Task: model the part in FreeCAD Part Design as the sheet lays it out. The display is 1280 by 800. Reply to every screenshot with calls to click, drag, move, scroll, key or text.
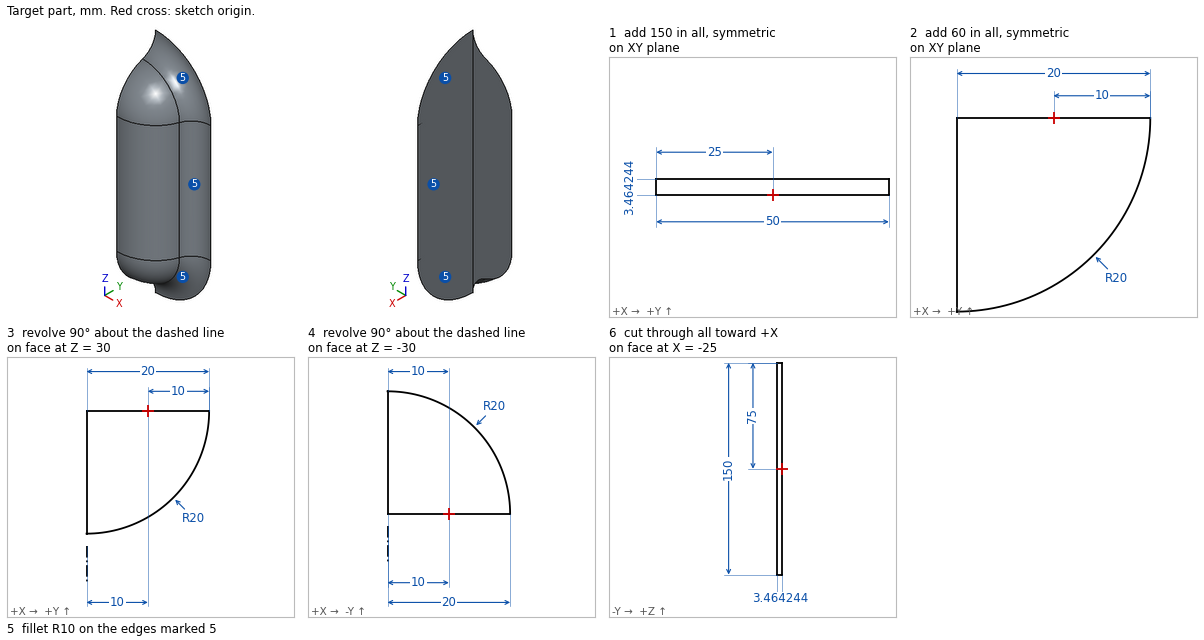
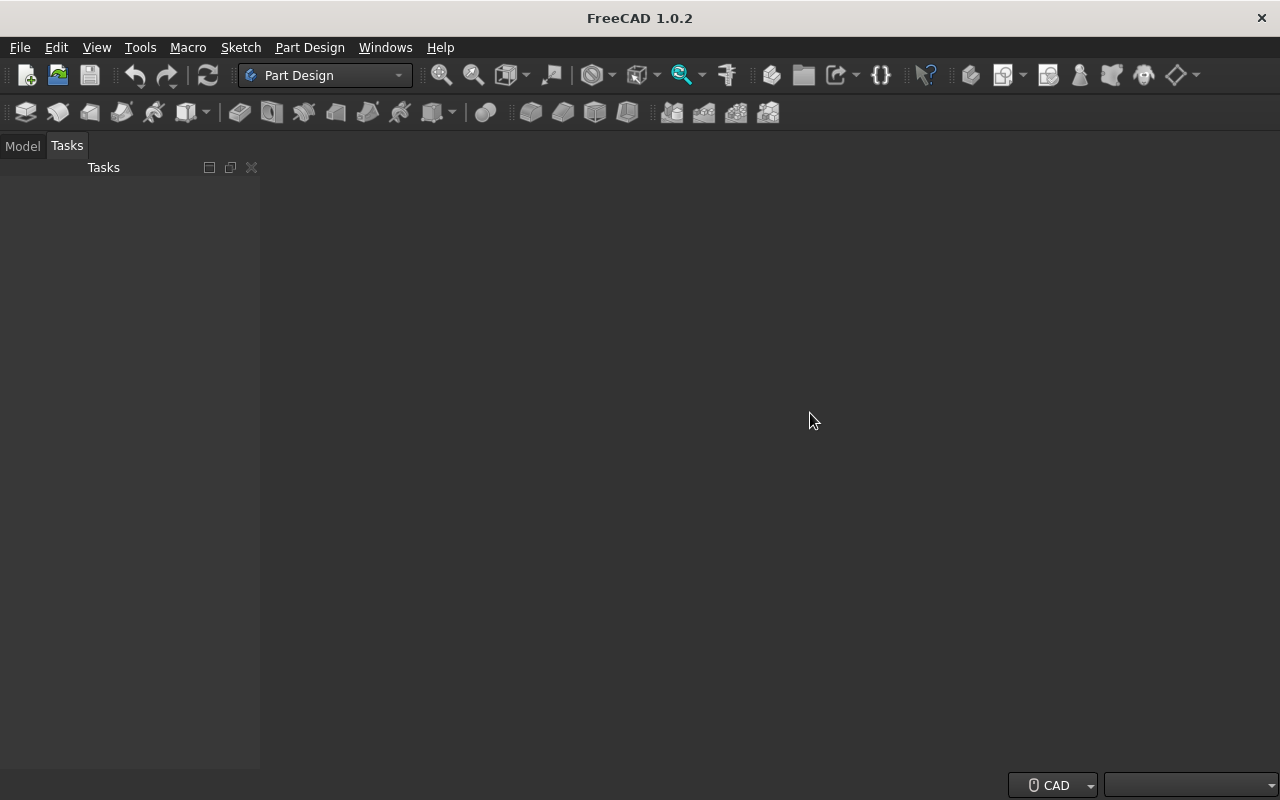
click(26, 76)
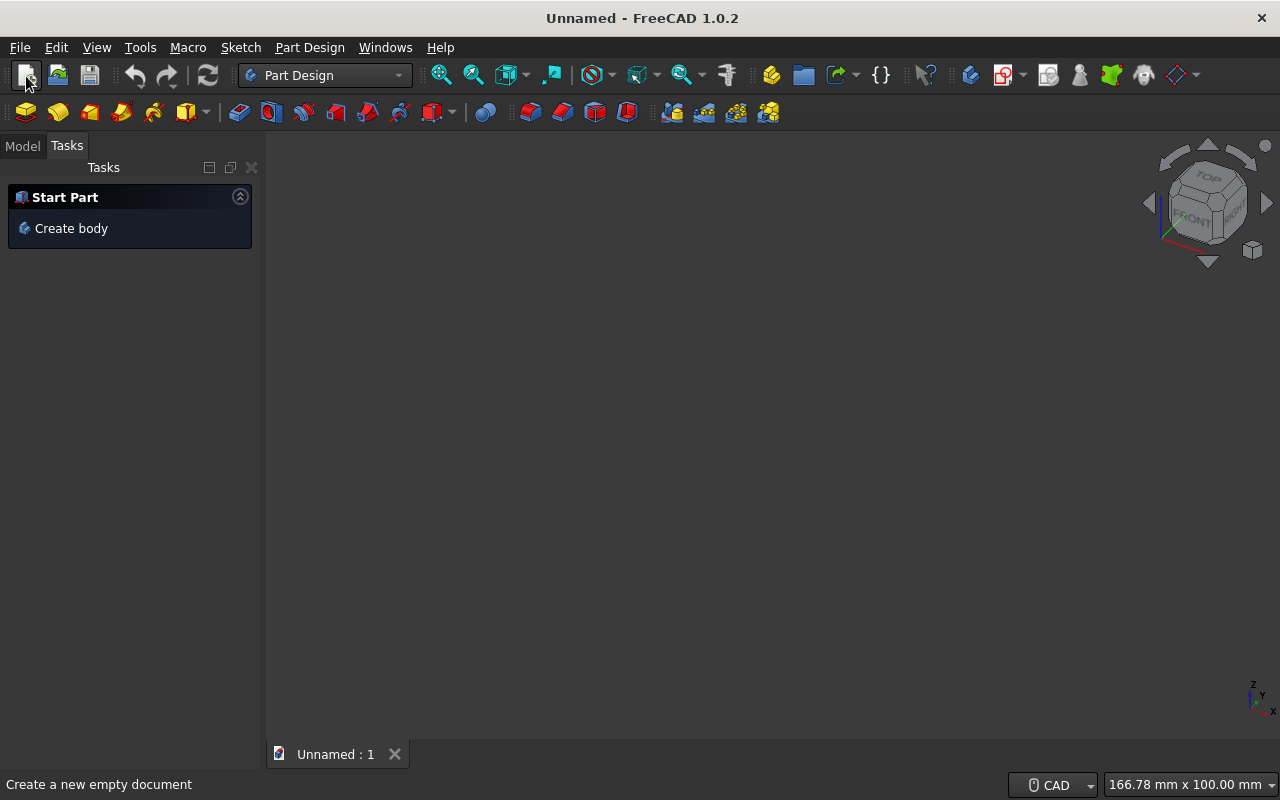
click(1004, 76)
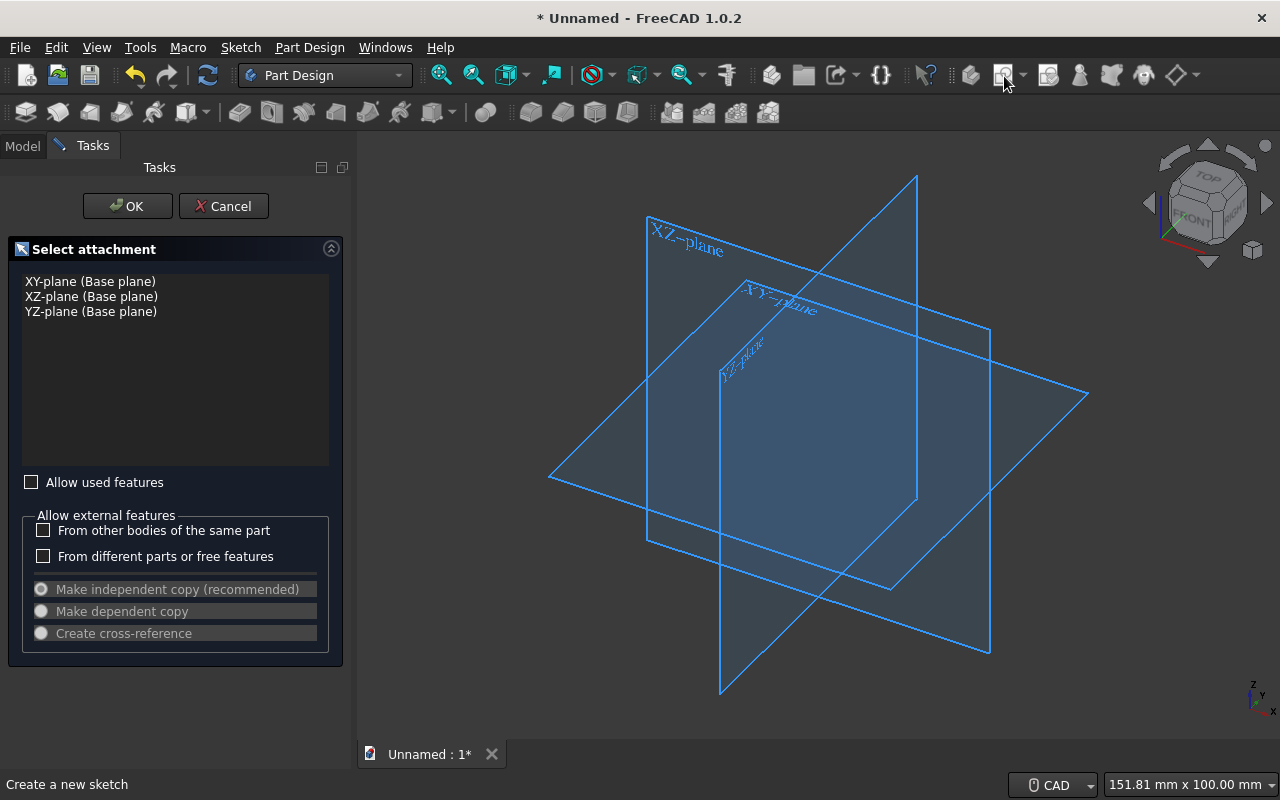
click(82, 282)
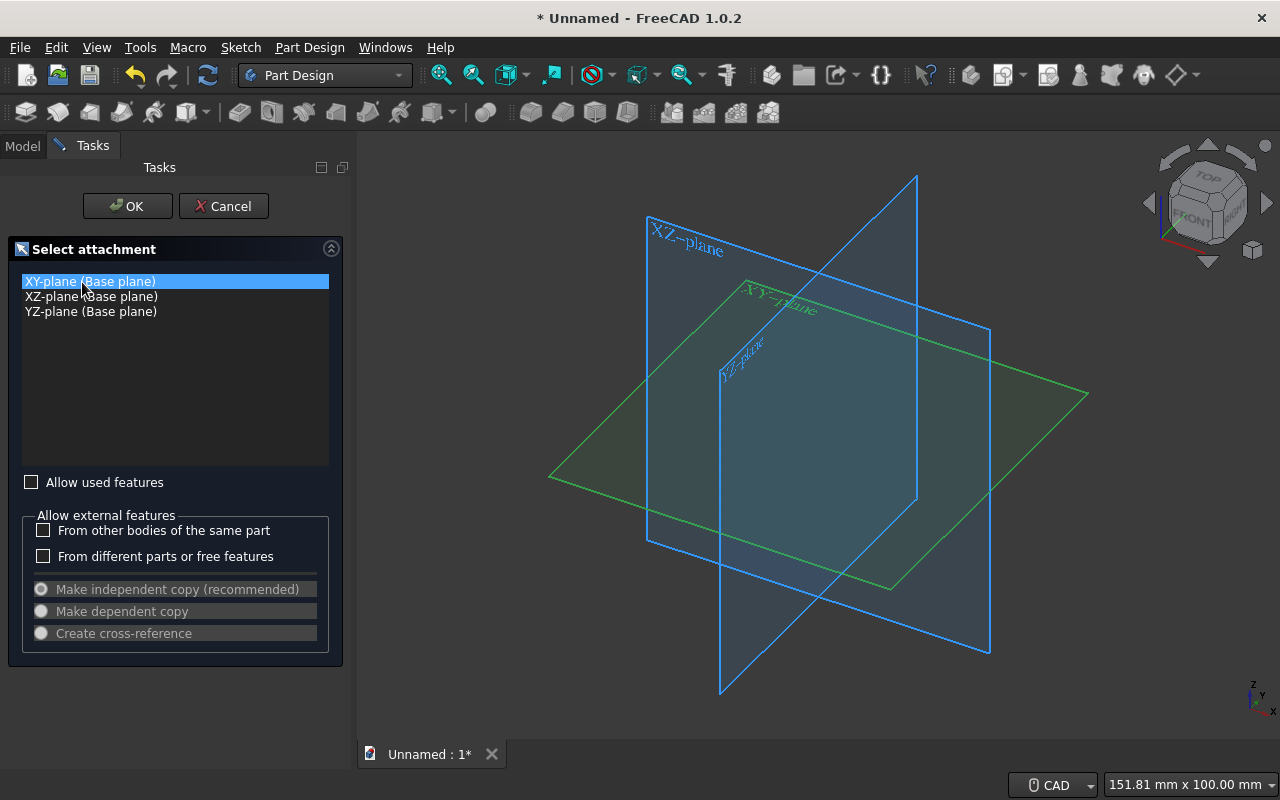
click(128, 206)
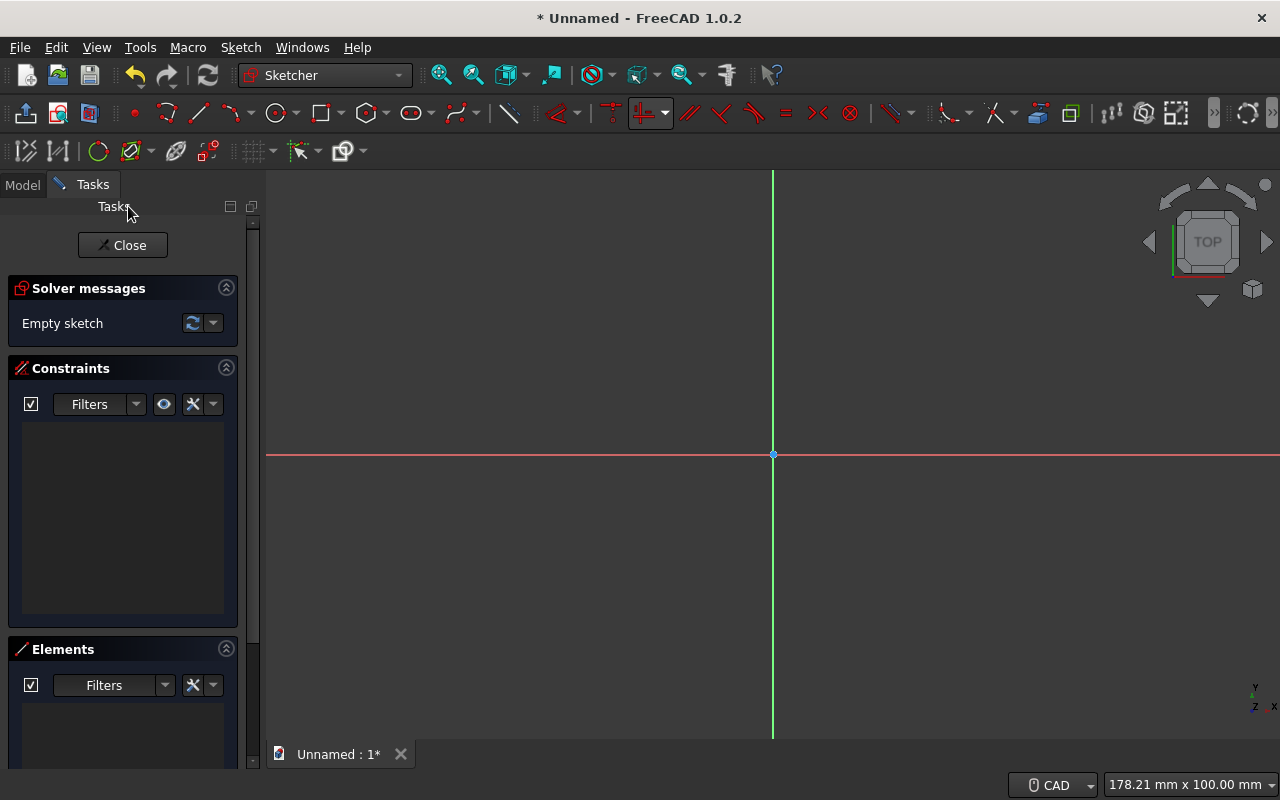
scroll(829, 437, up, 4)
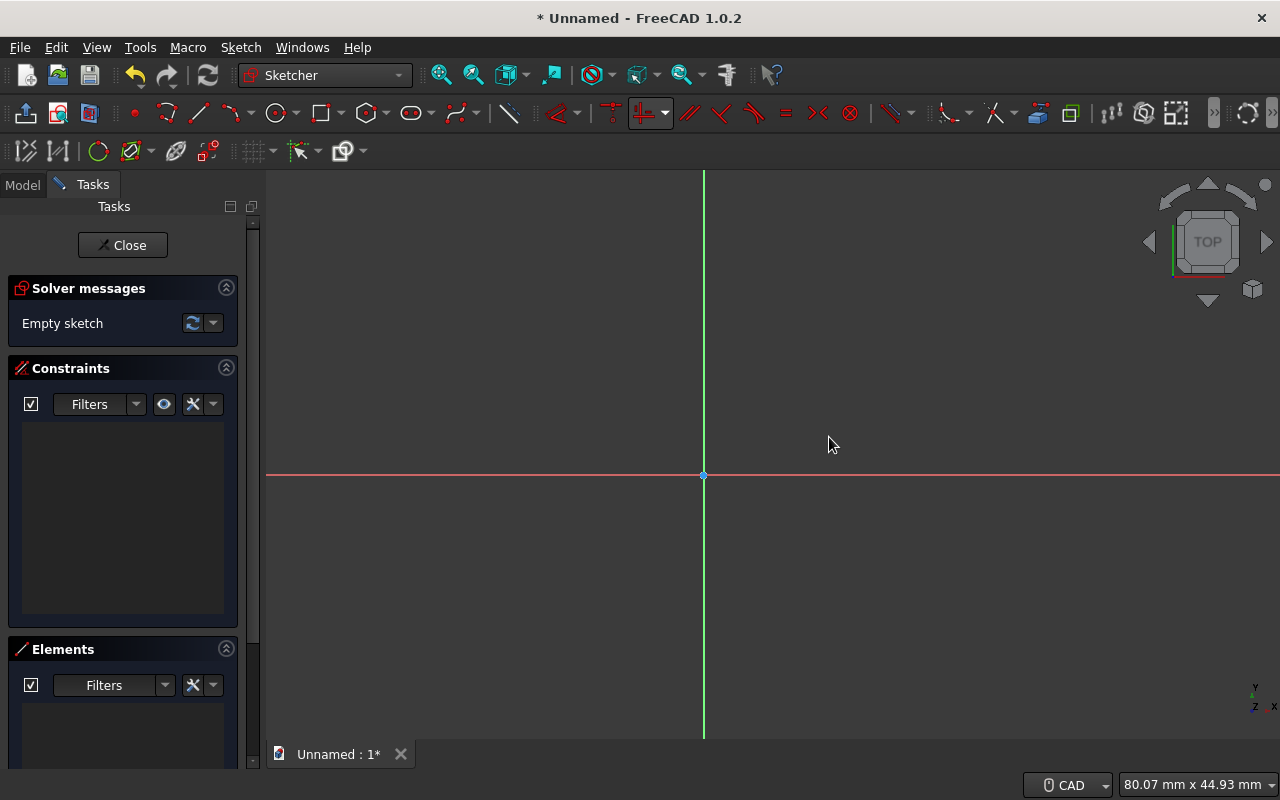
click(322, 114)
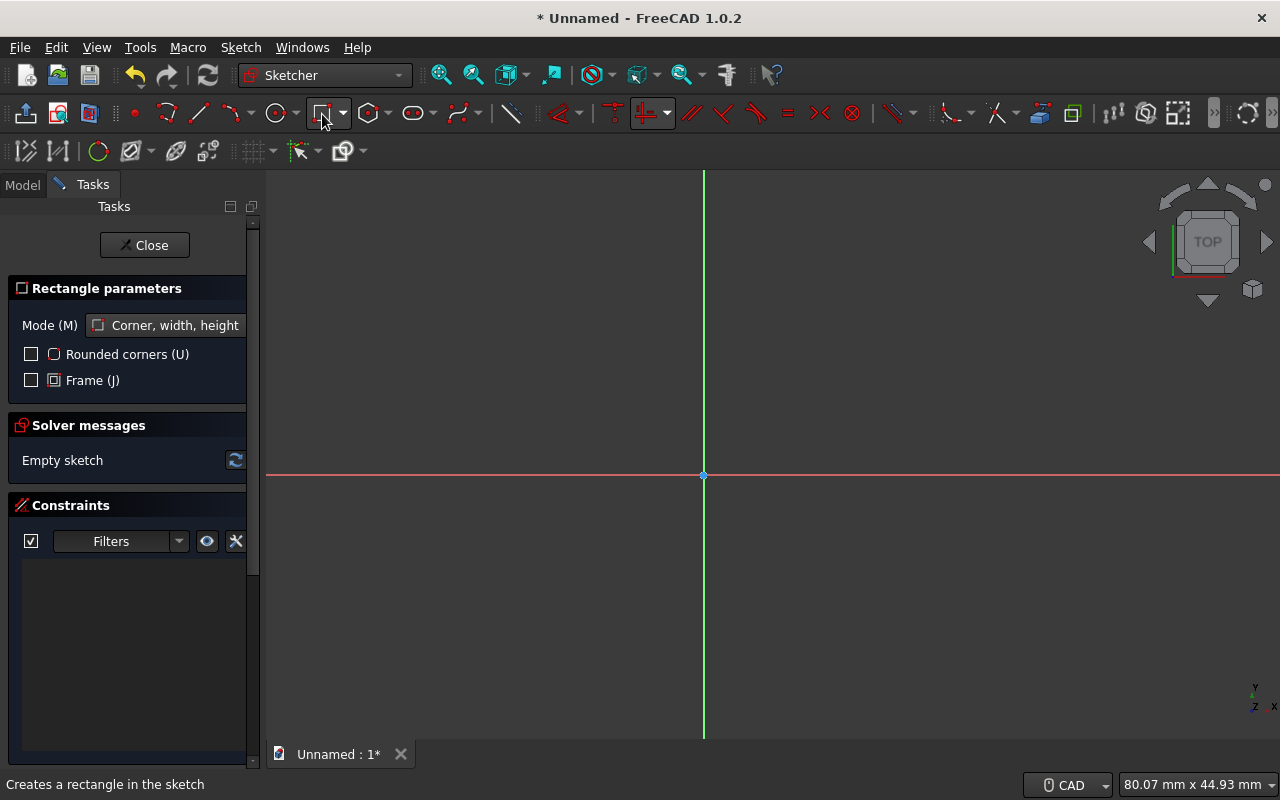
click(387, 432)
click(1020, 475)
key(Escape)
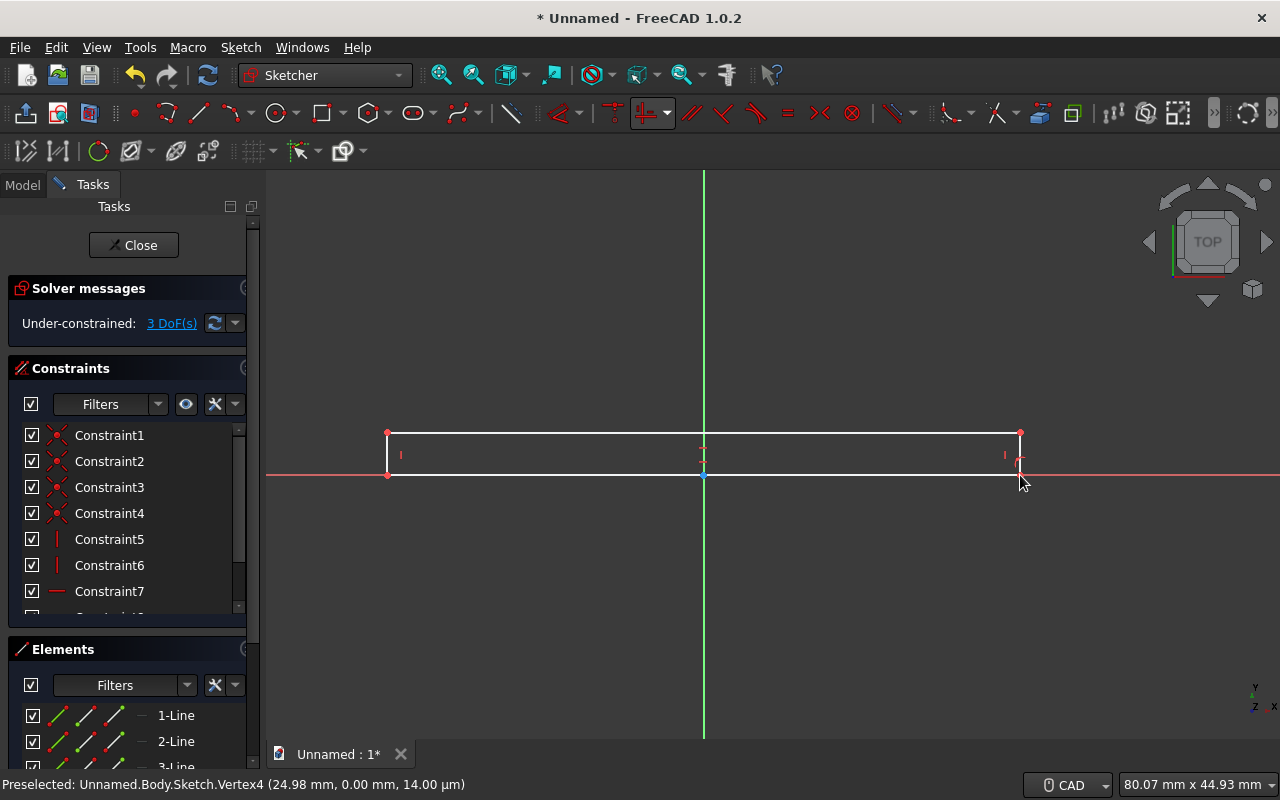
click(558, 114)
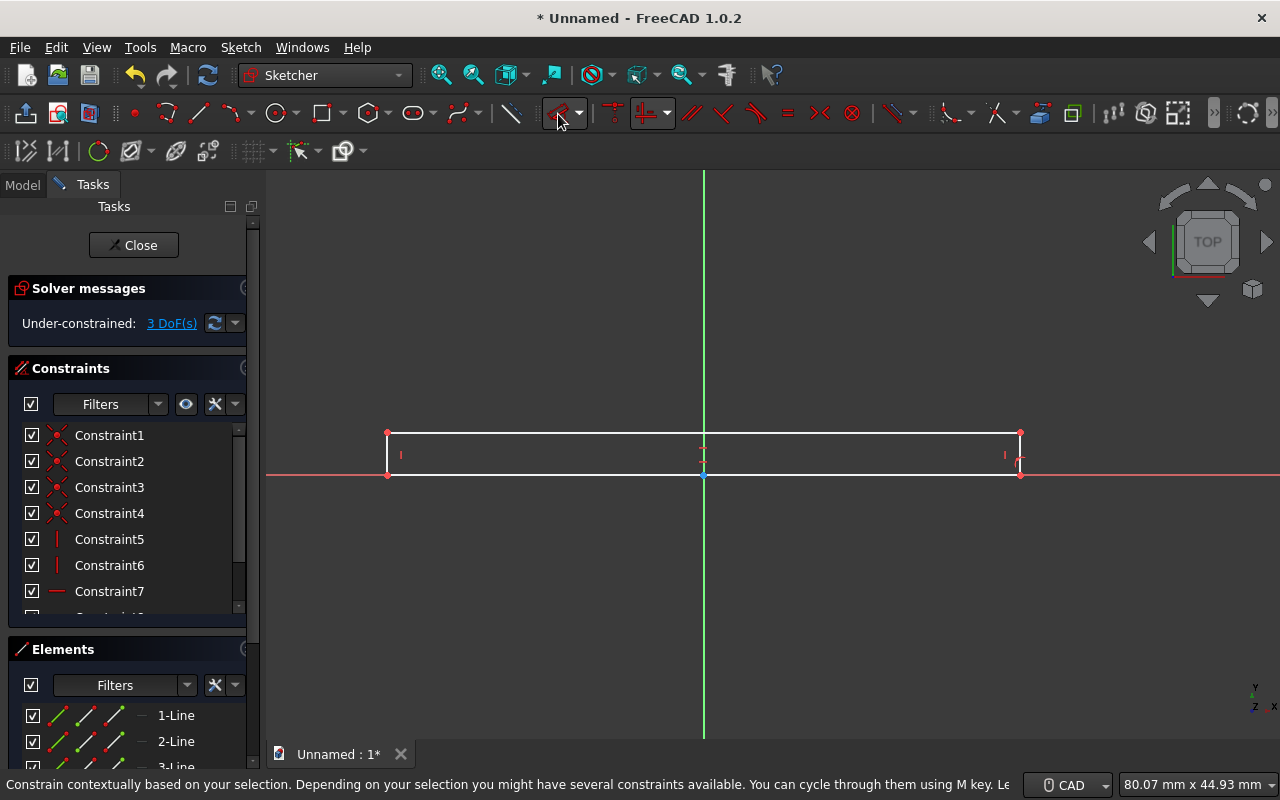
click(577, 475)
click(558, 509)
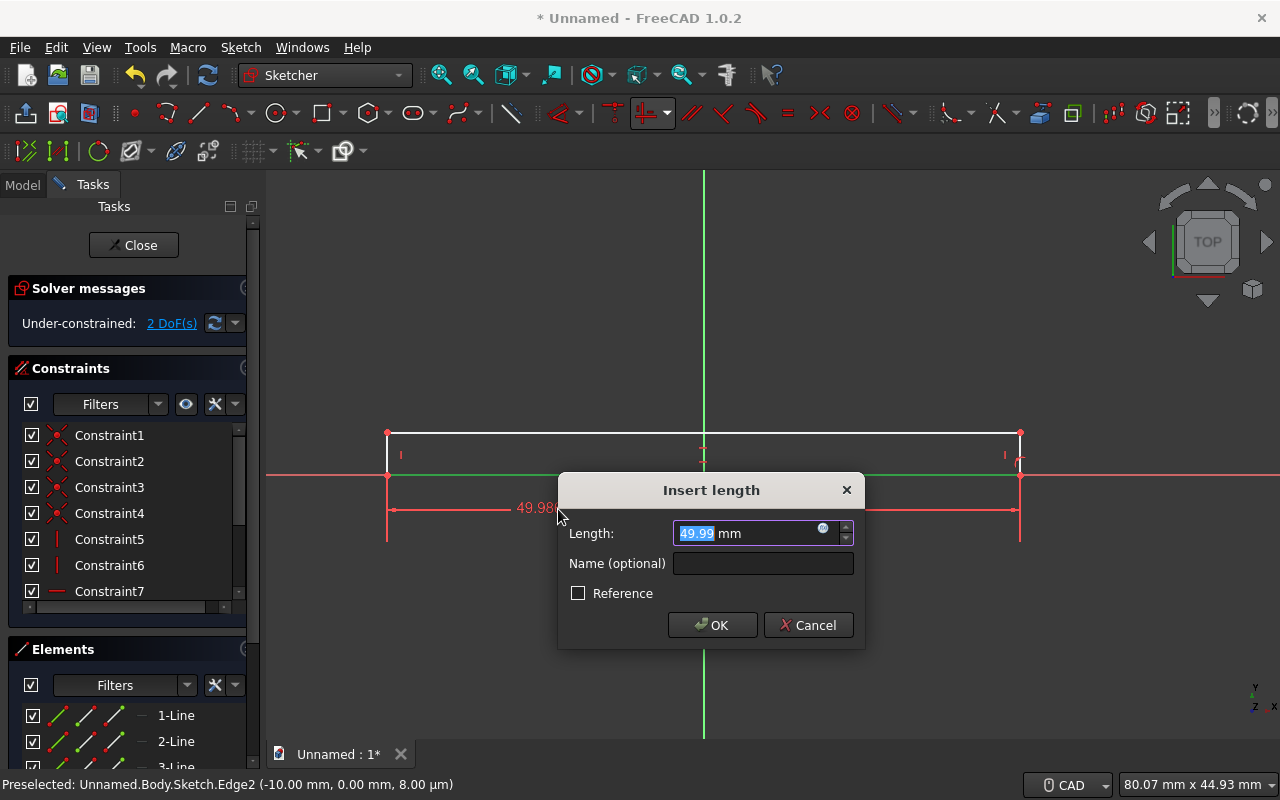
text(50)
key(Return)